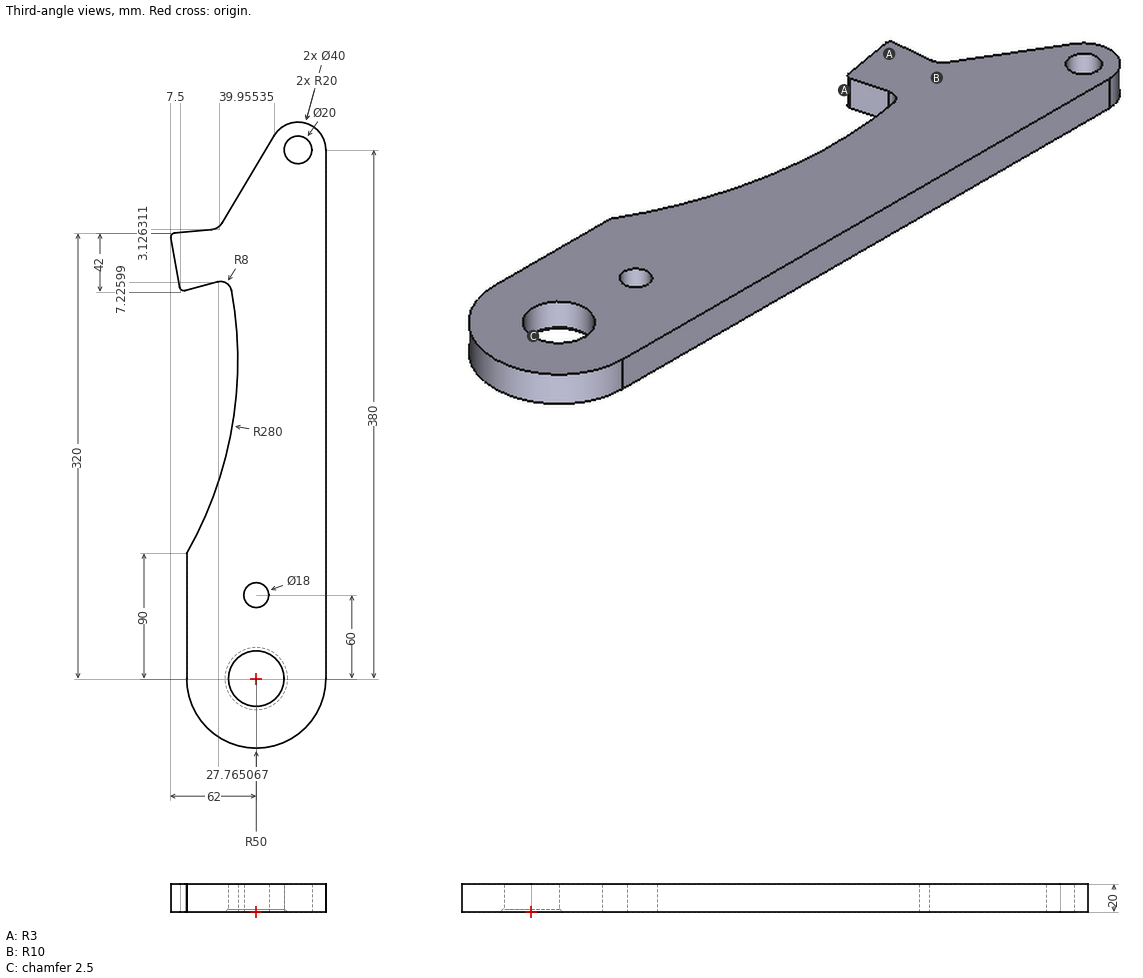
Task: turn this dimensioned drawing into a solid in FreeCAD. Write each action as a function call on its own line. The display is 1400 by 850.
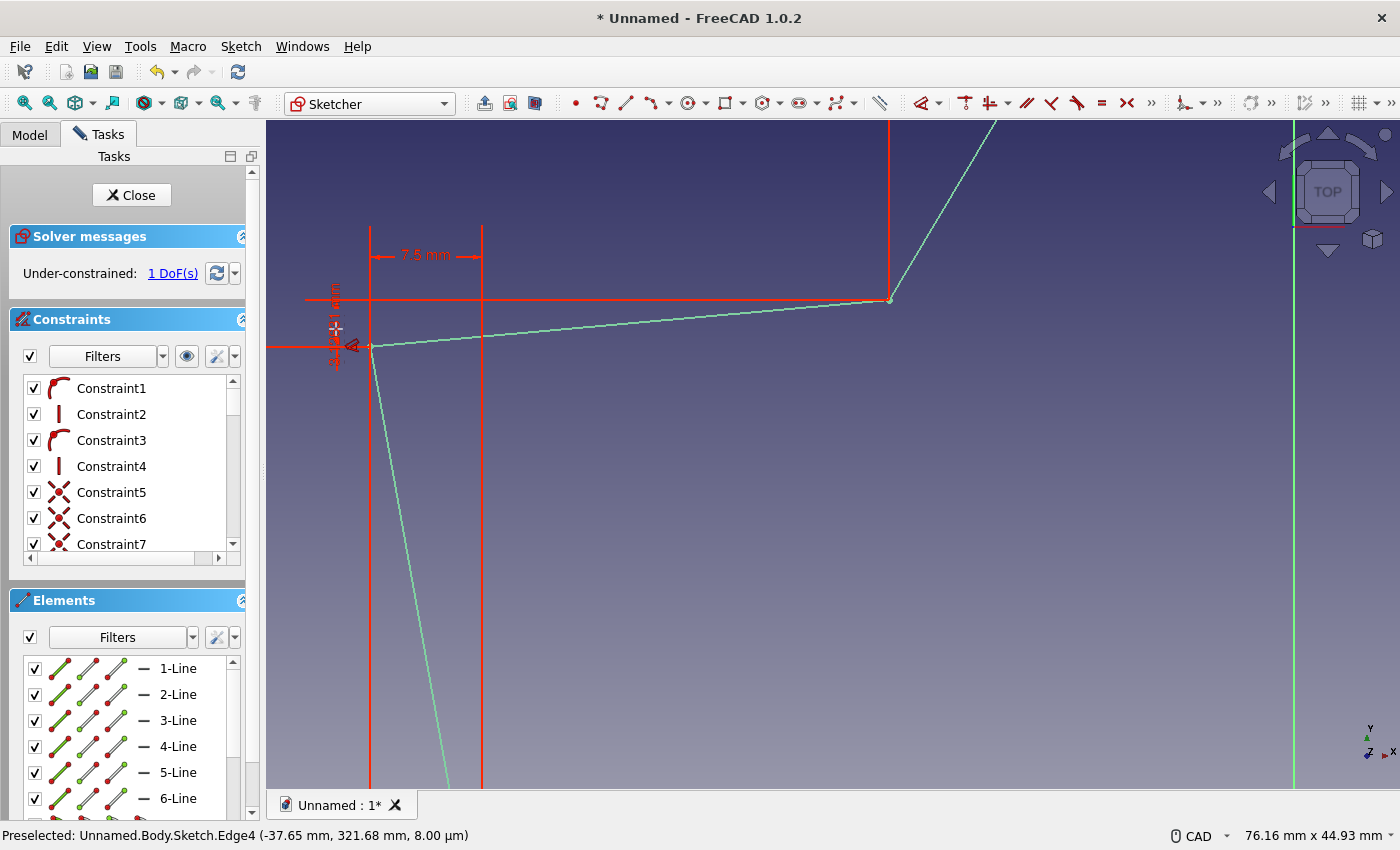
scroll(736, 321, down, 14)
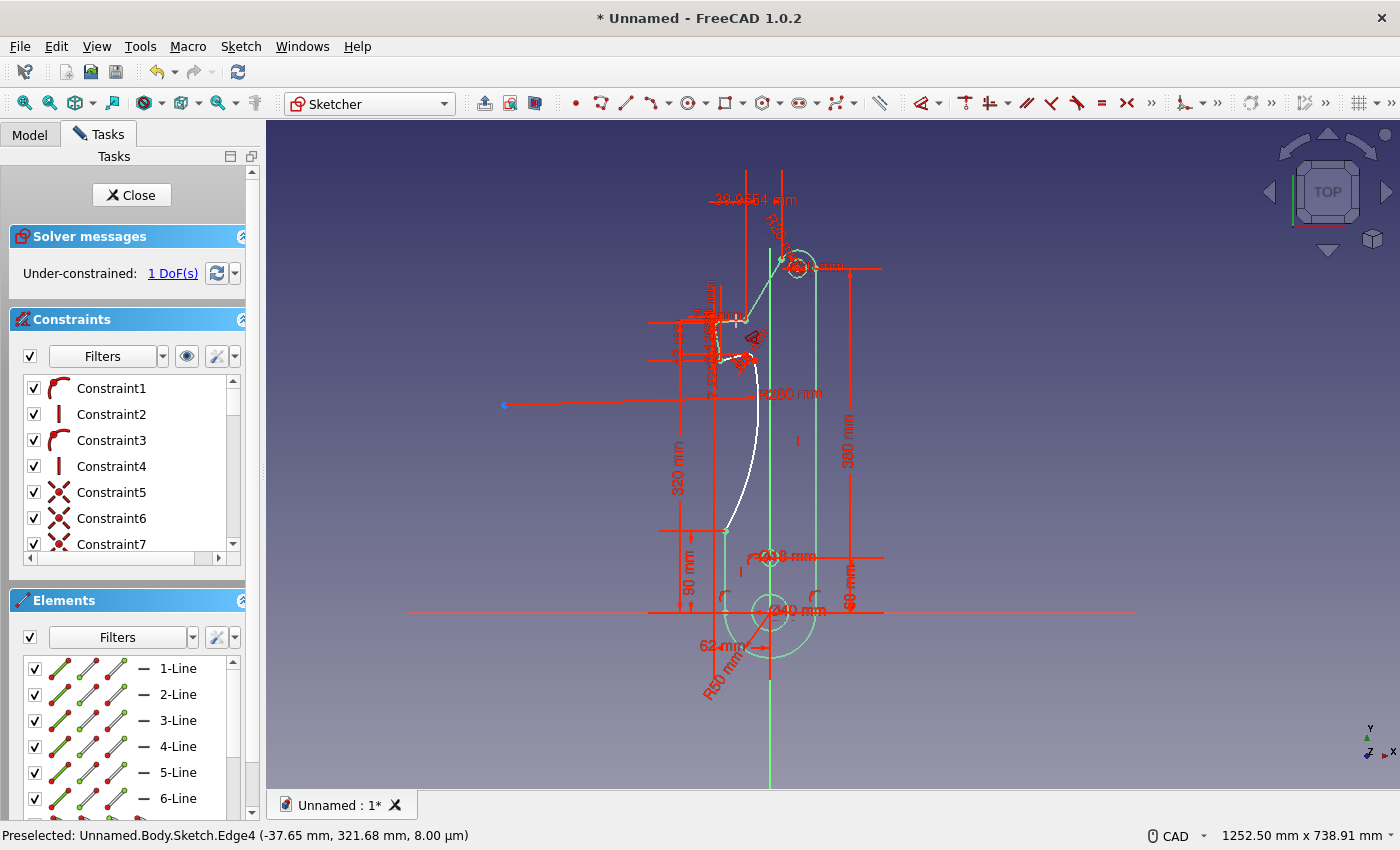
scroll(745, 354, up, 3)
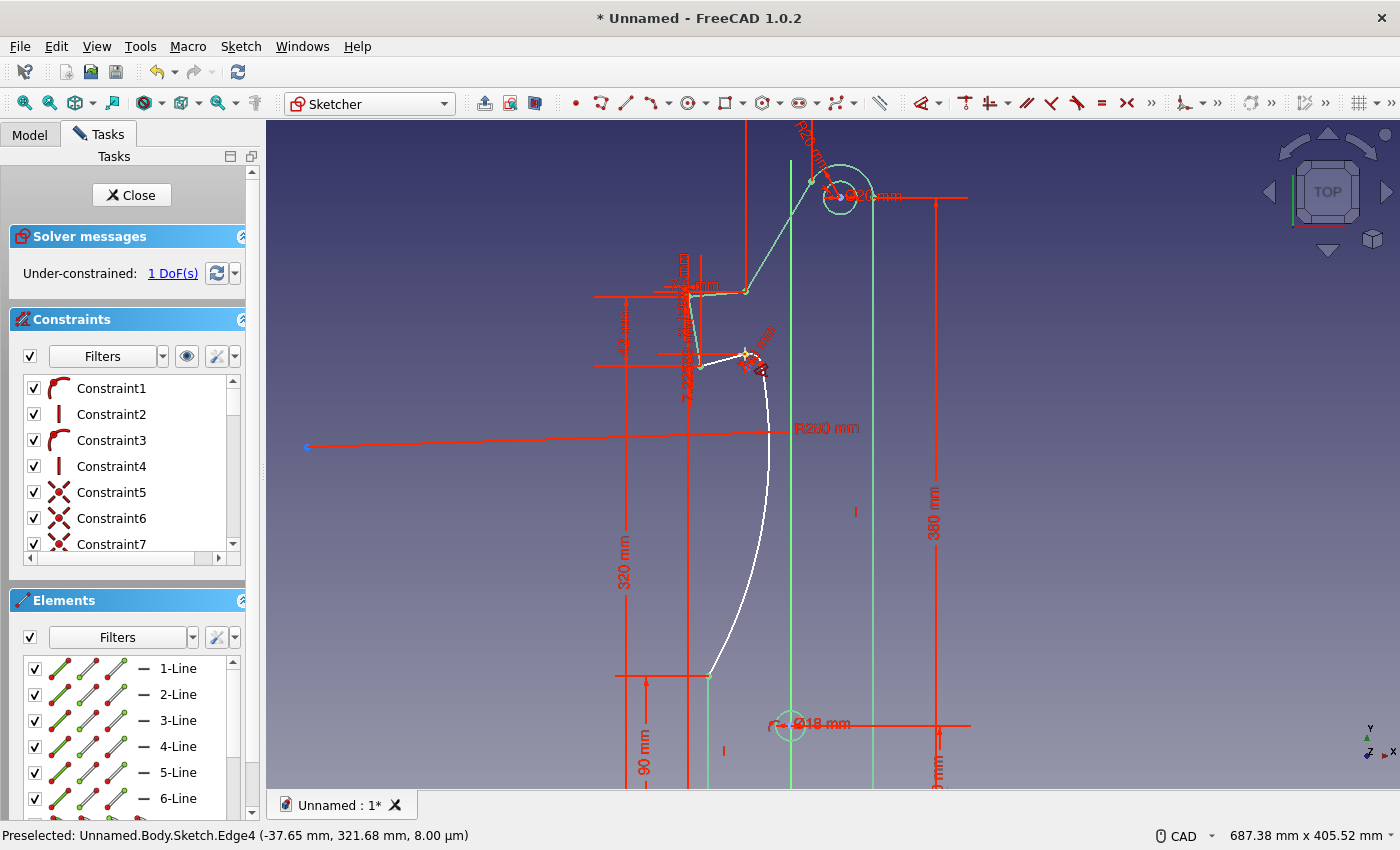
click(745, 354)
click(768, 320)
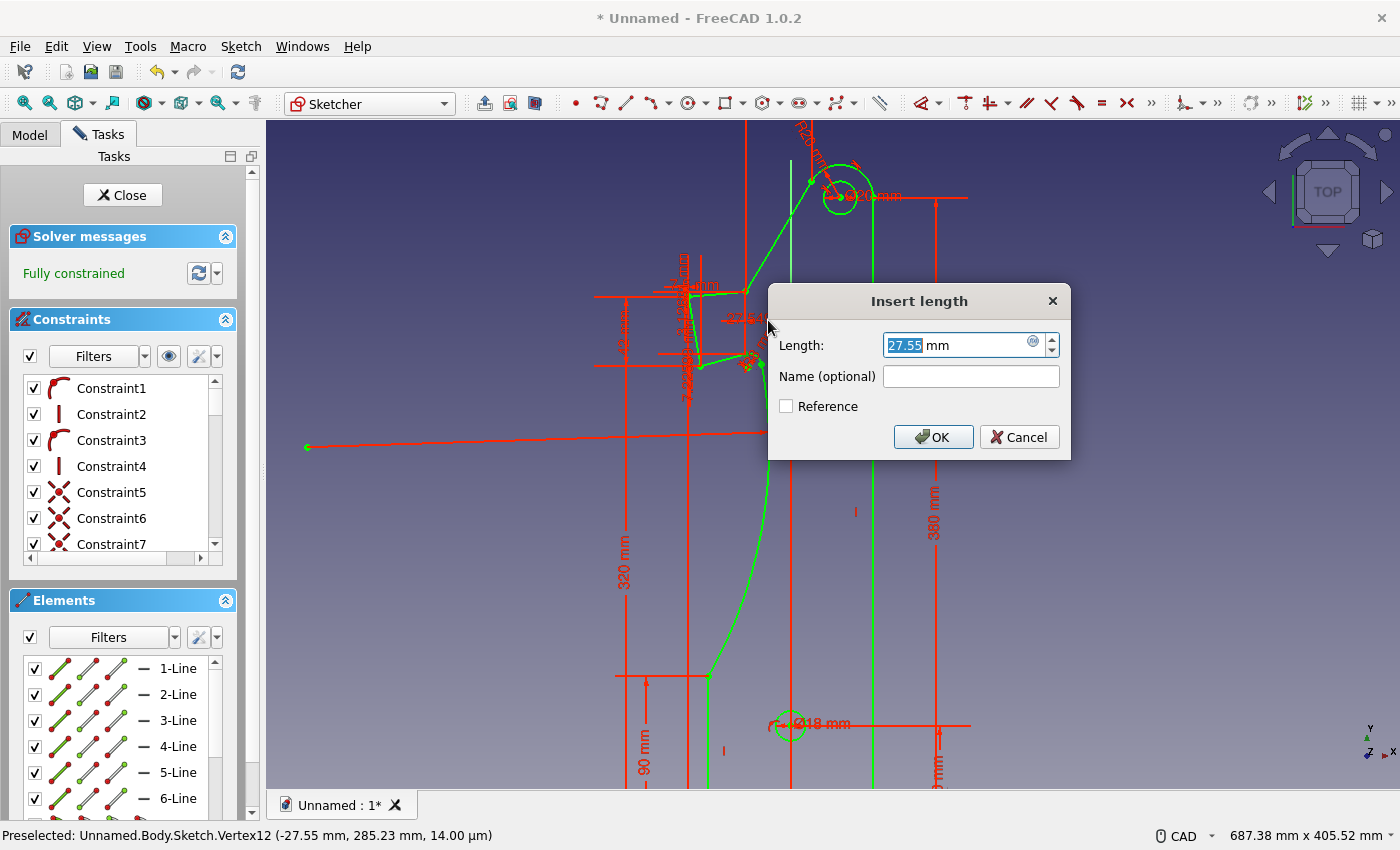
text(27.765067)
key(Return)
key(Escape)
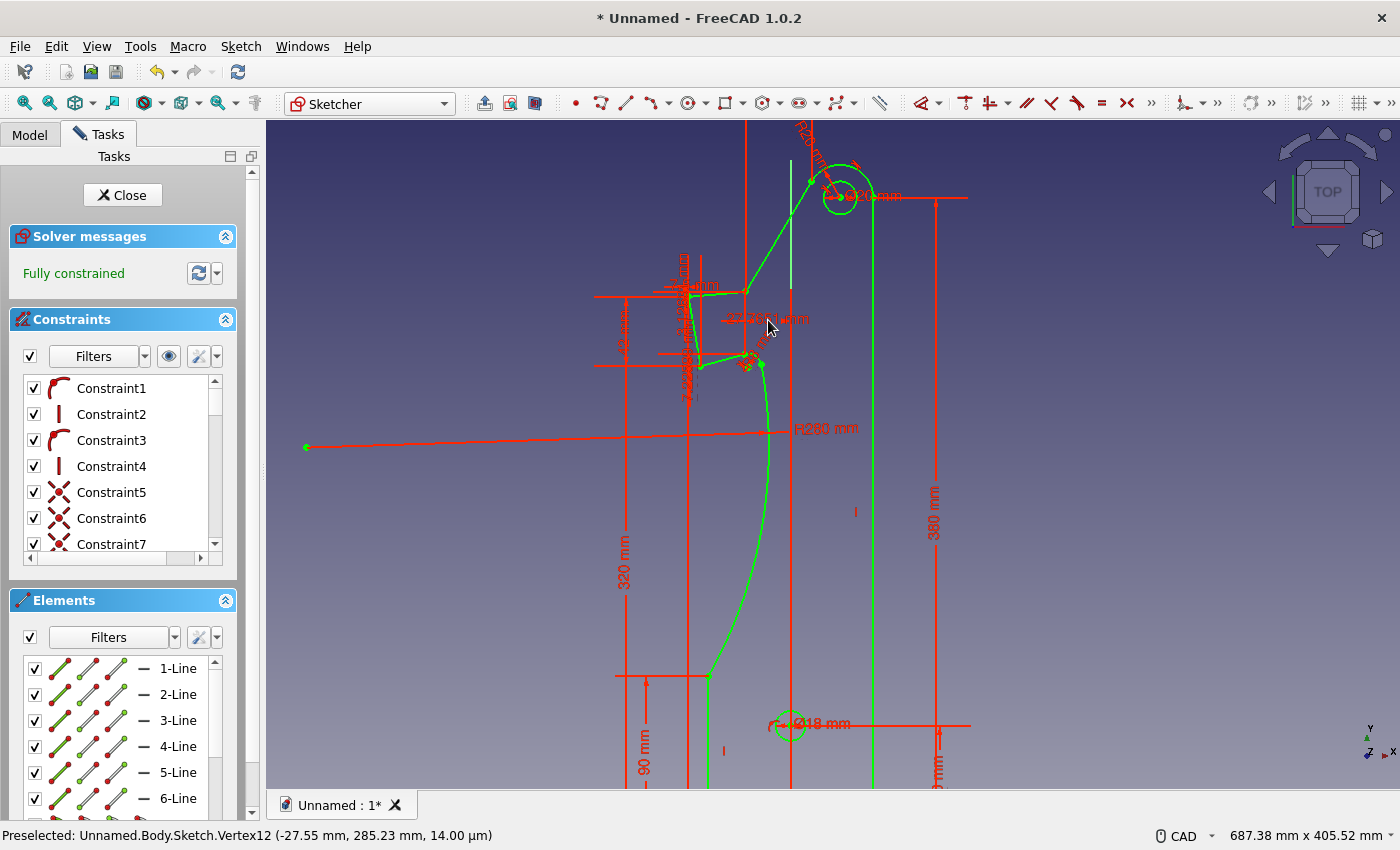
click(123, 195)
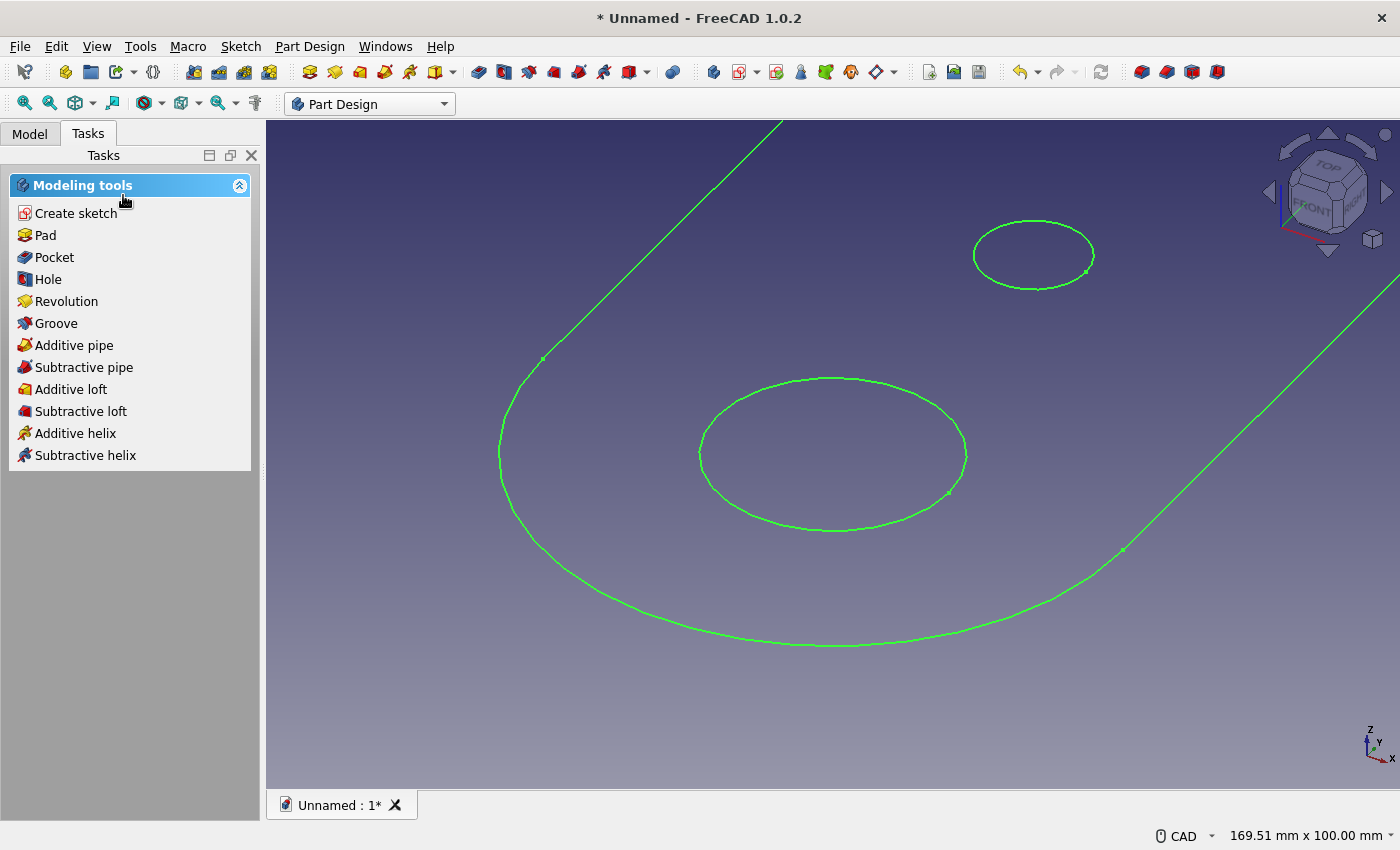
click(310, 72)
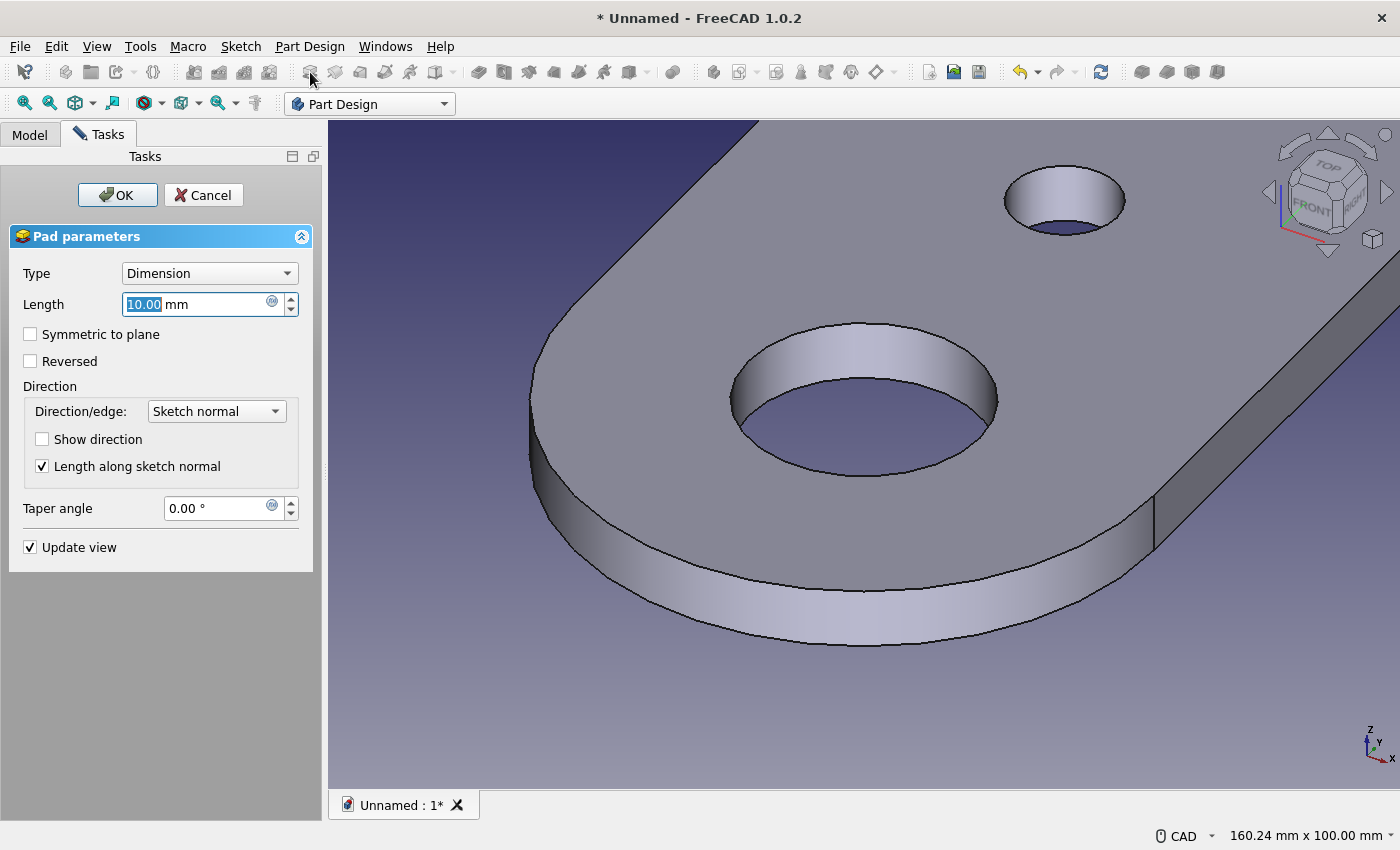
text(20)
key(Tab)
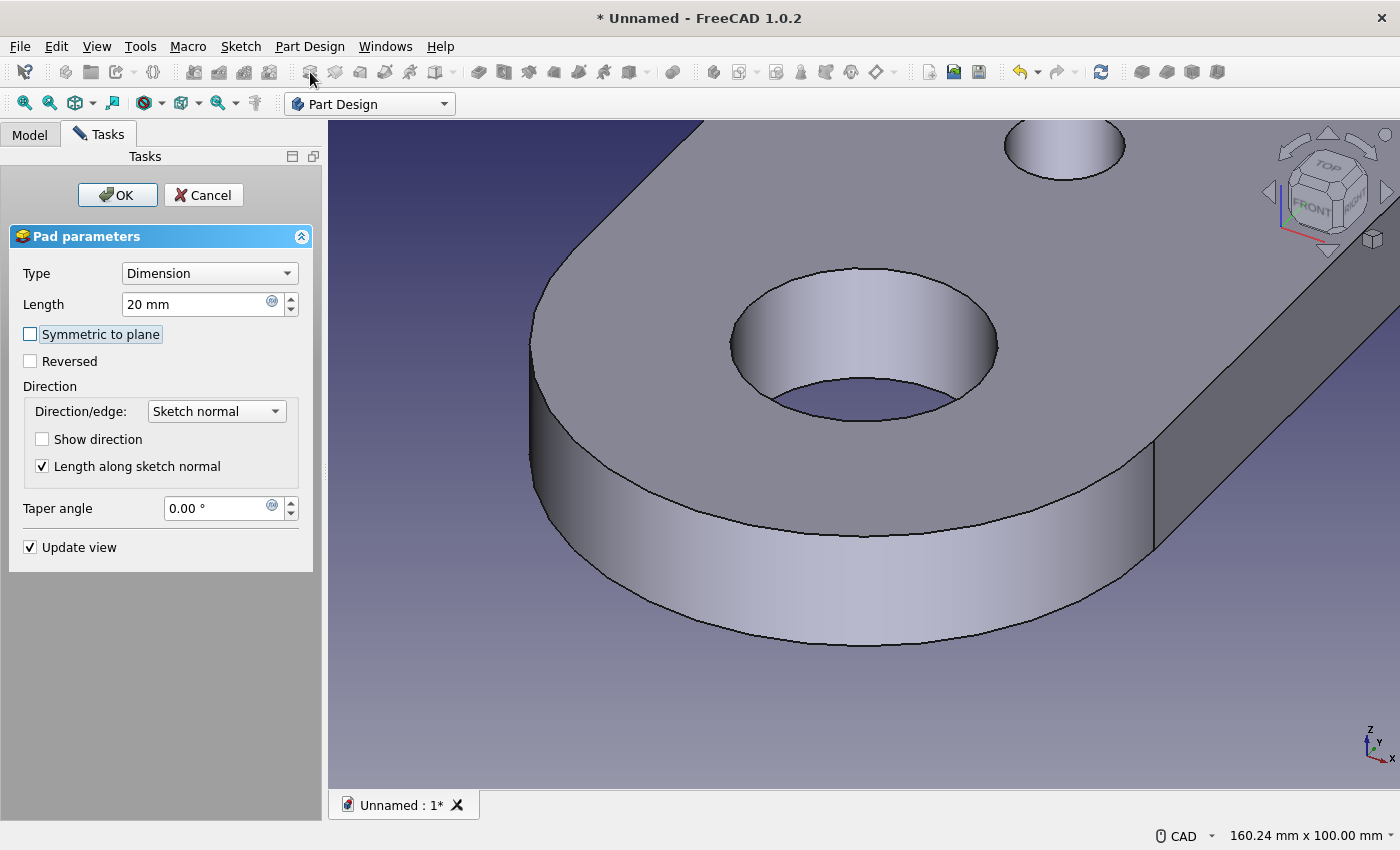
click(118, 195)